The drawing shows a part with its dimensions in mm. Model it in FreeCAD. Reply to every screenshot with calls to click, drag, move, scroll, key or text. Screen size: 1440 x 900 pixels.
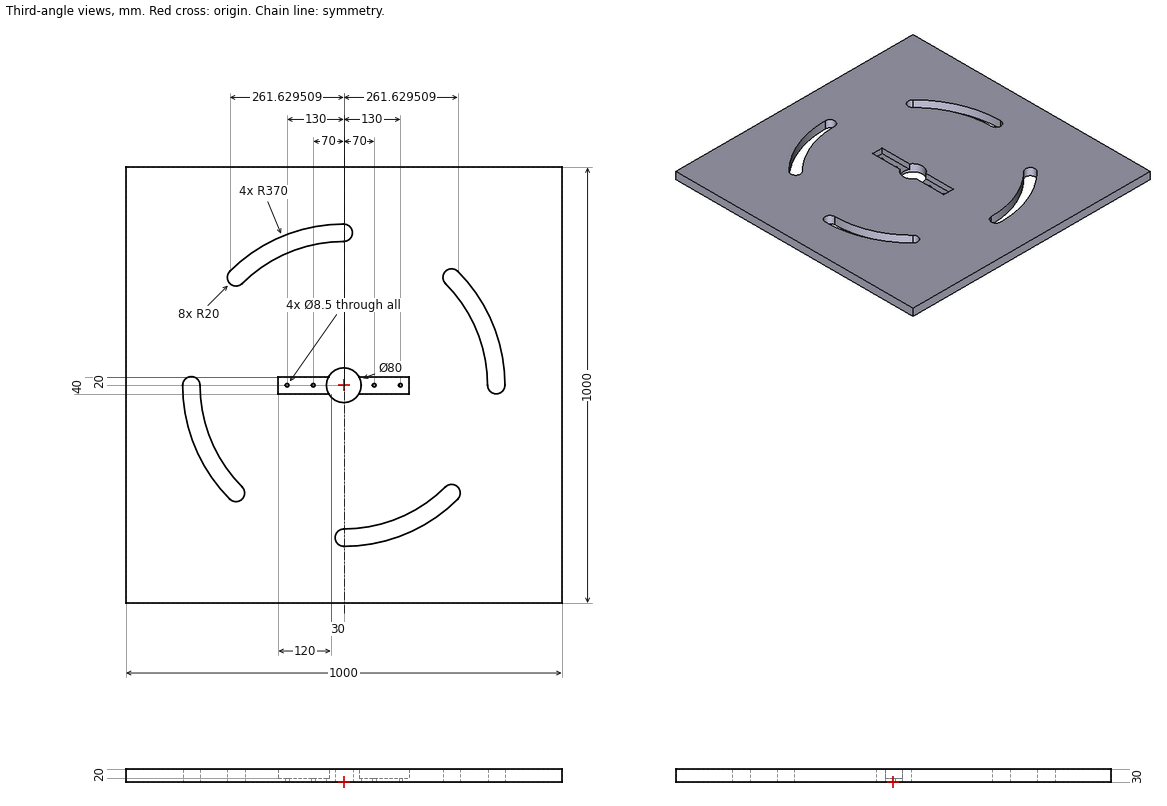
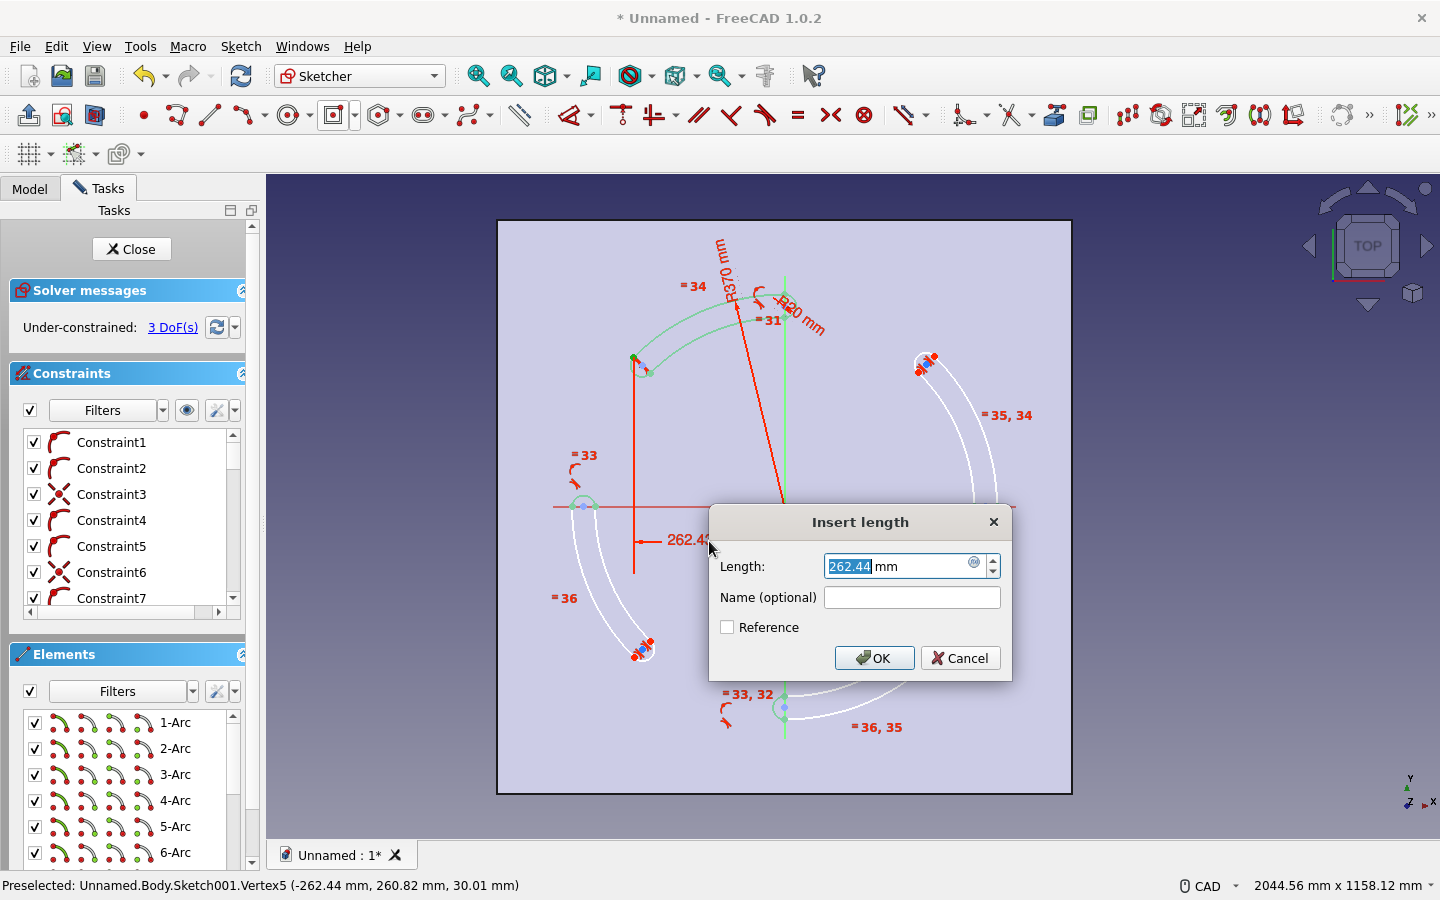
text(261.629509)
key(Return)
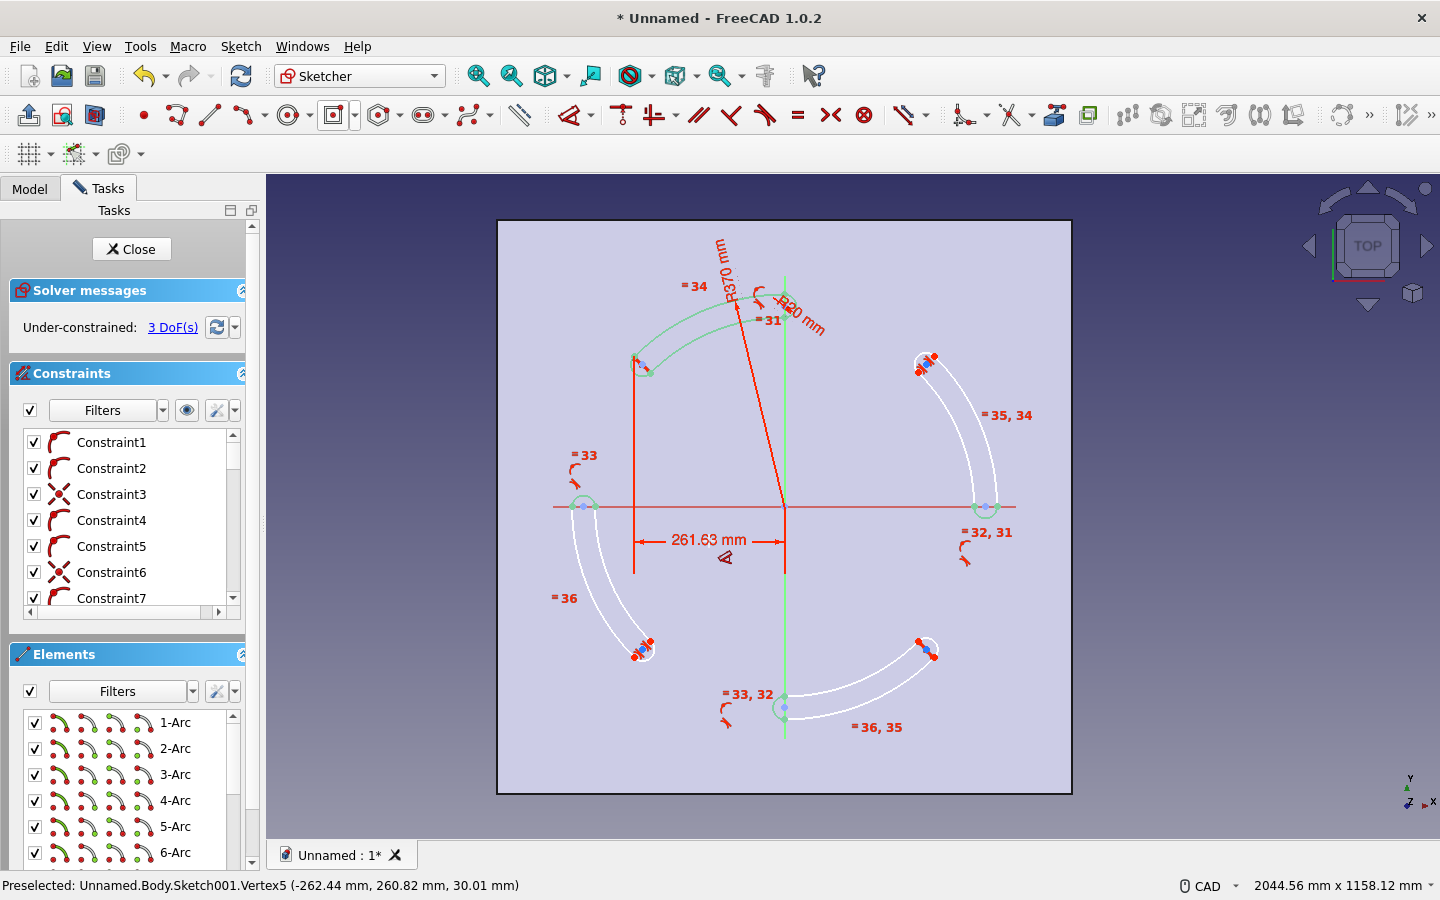
click(934, 356)
click(894, 322)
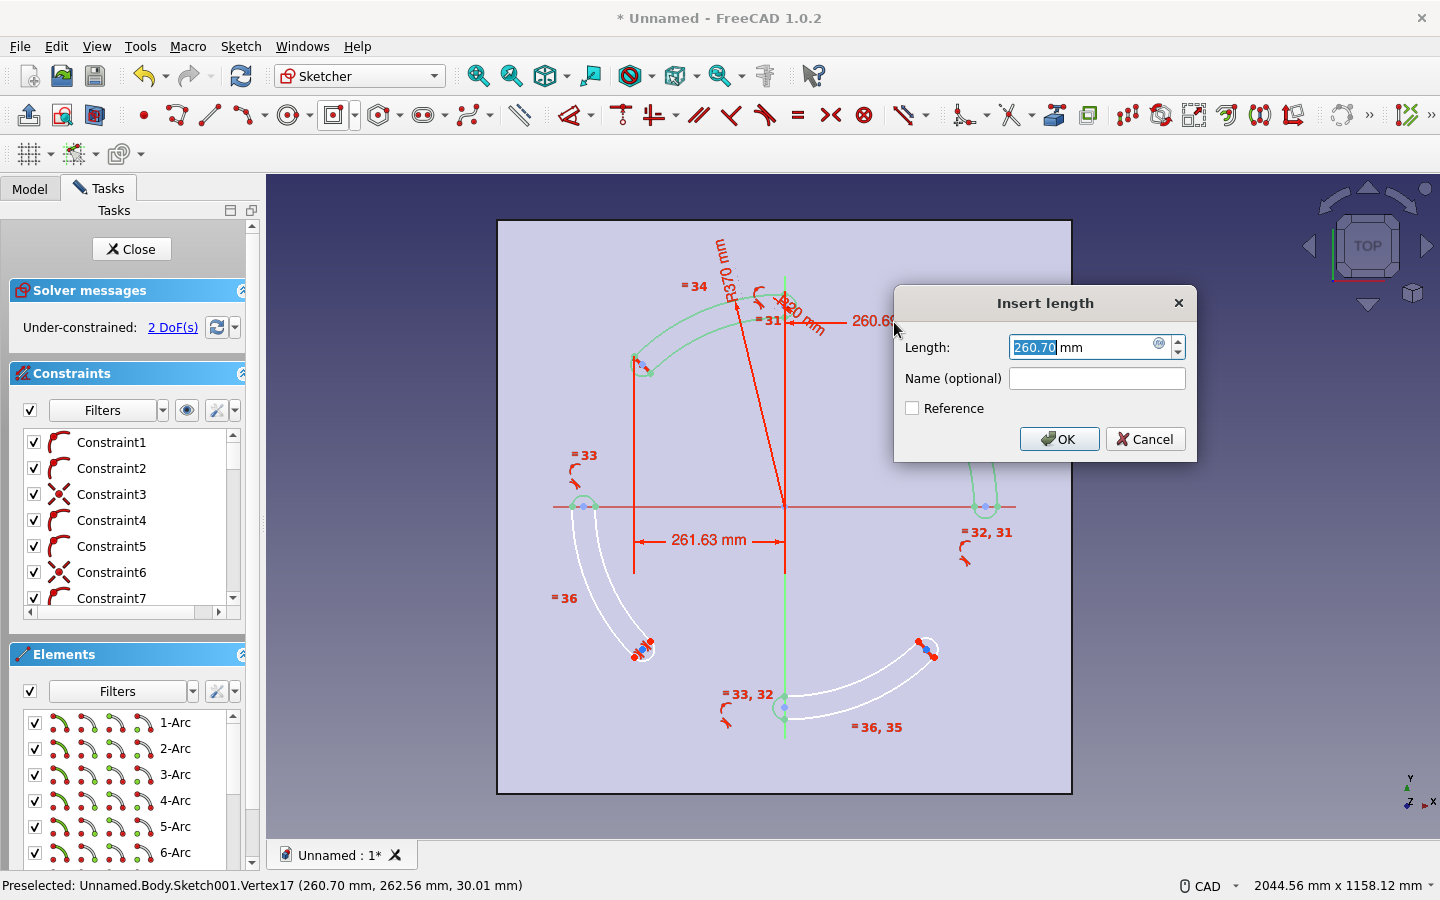
text(261.629509)
key(Return)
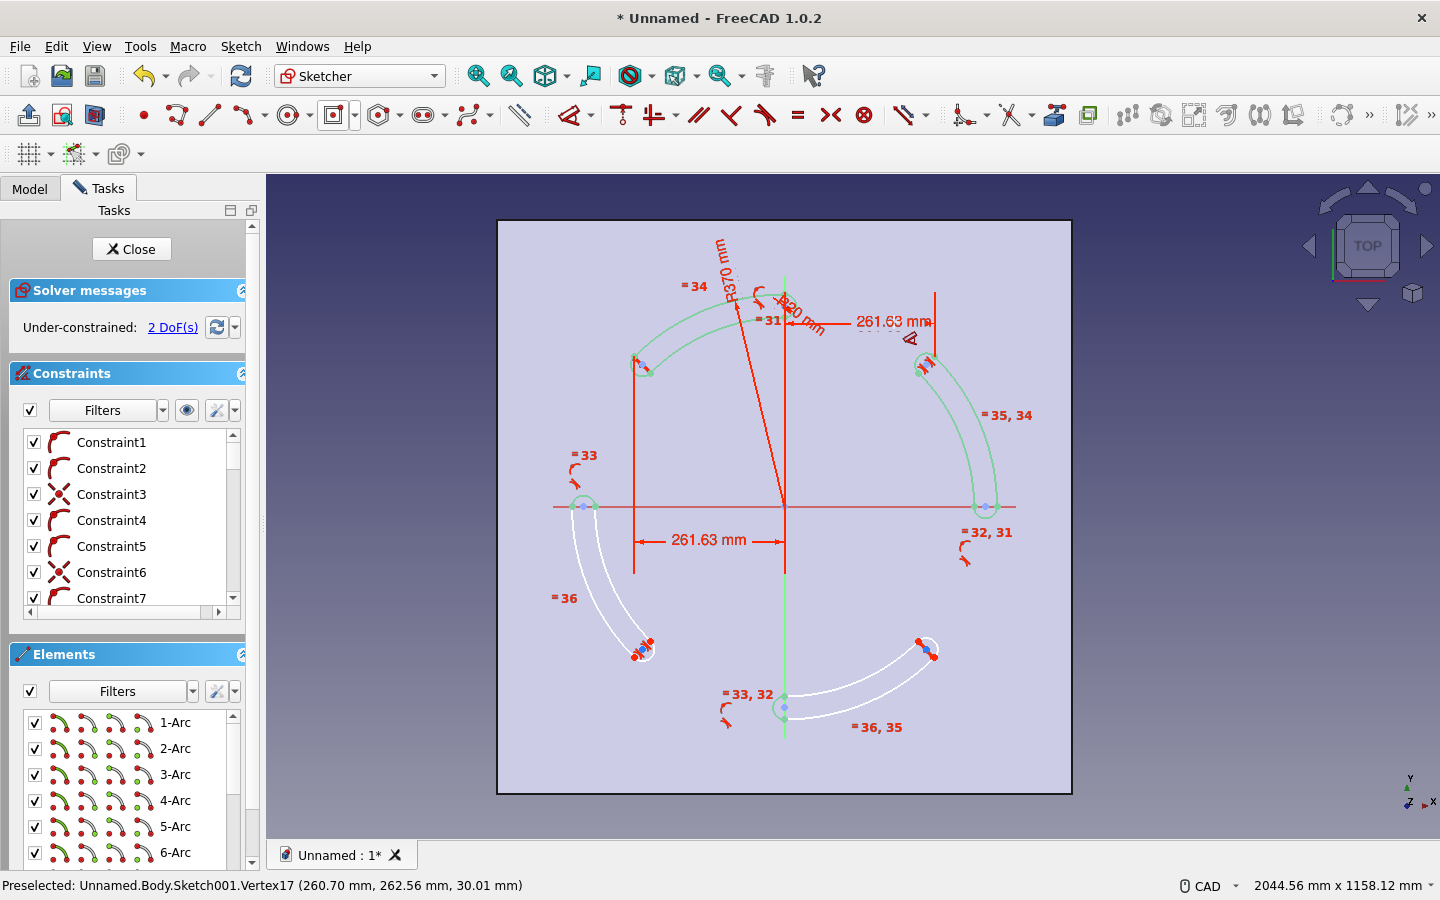
click(934, 658)
click(859, 473)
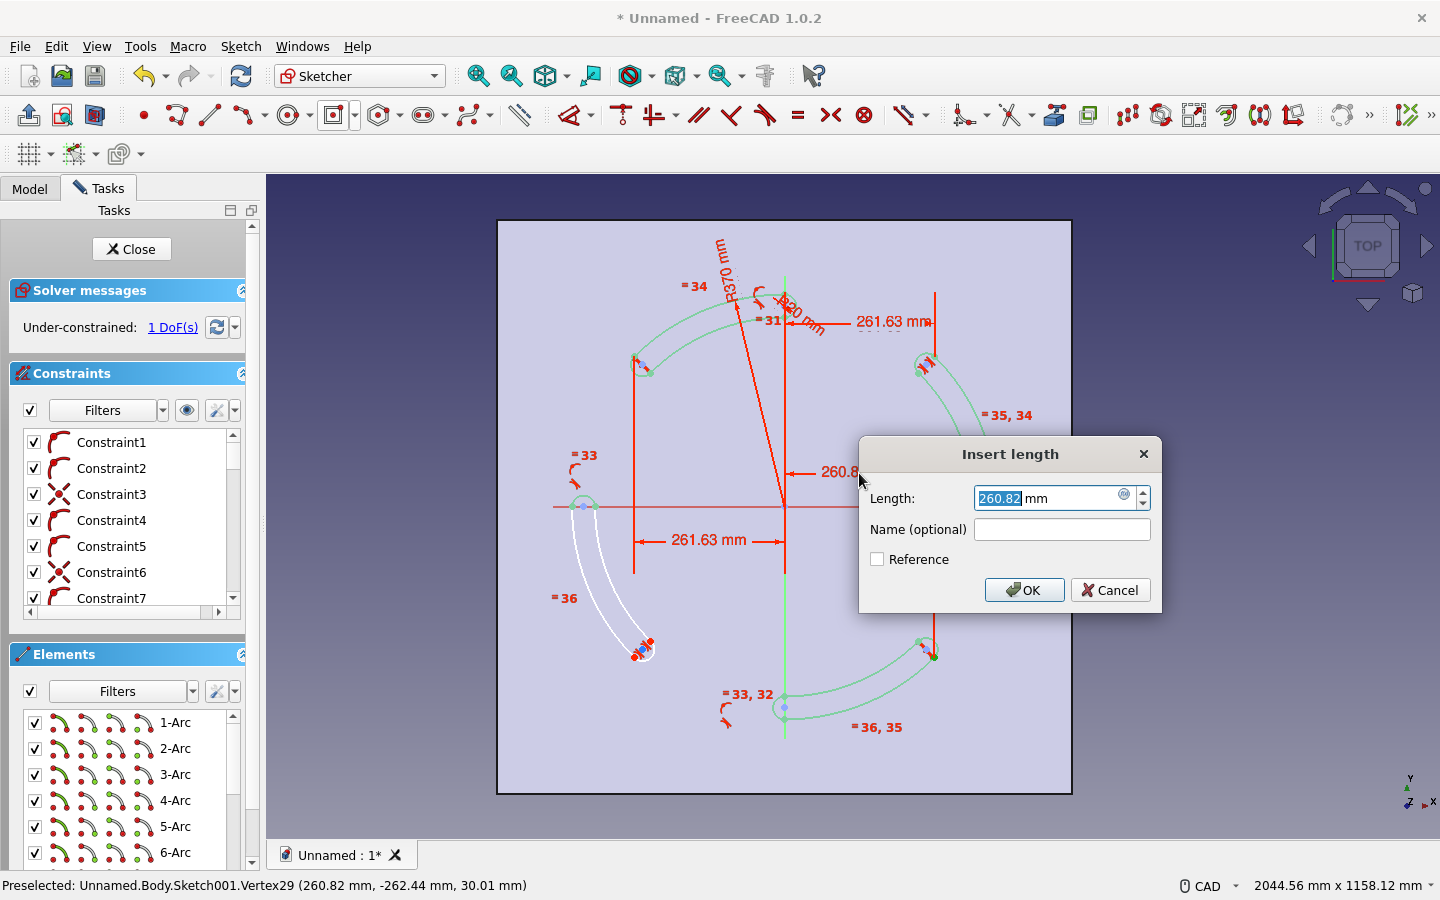
text(261.629509)
key(Return)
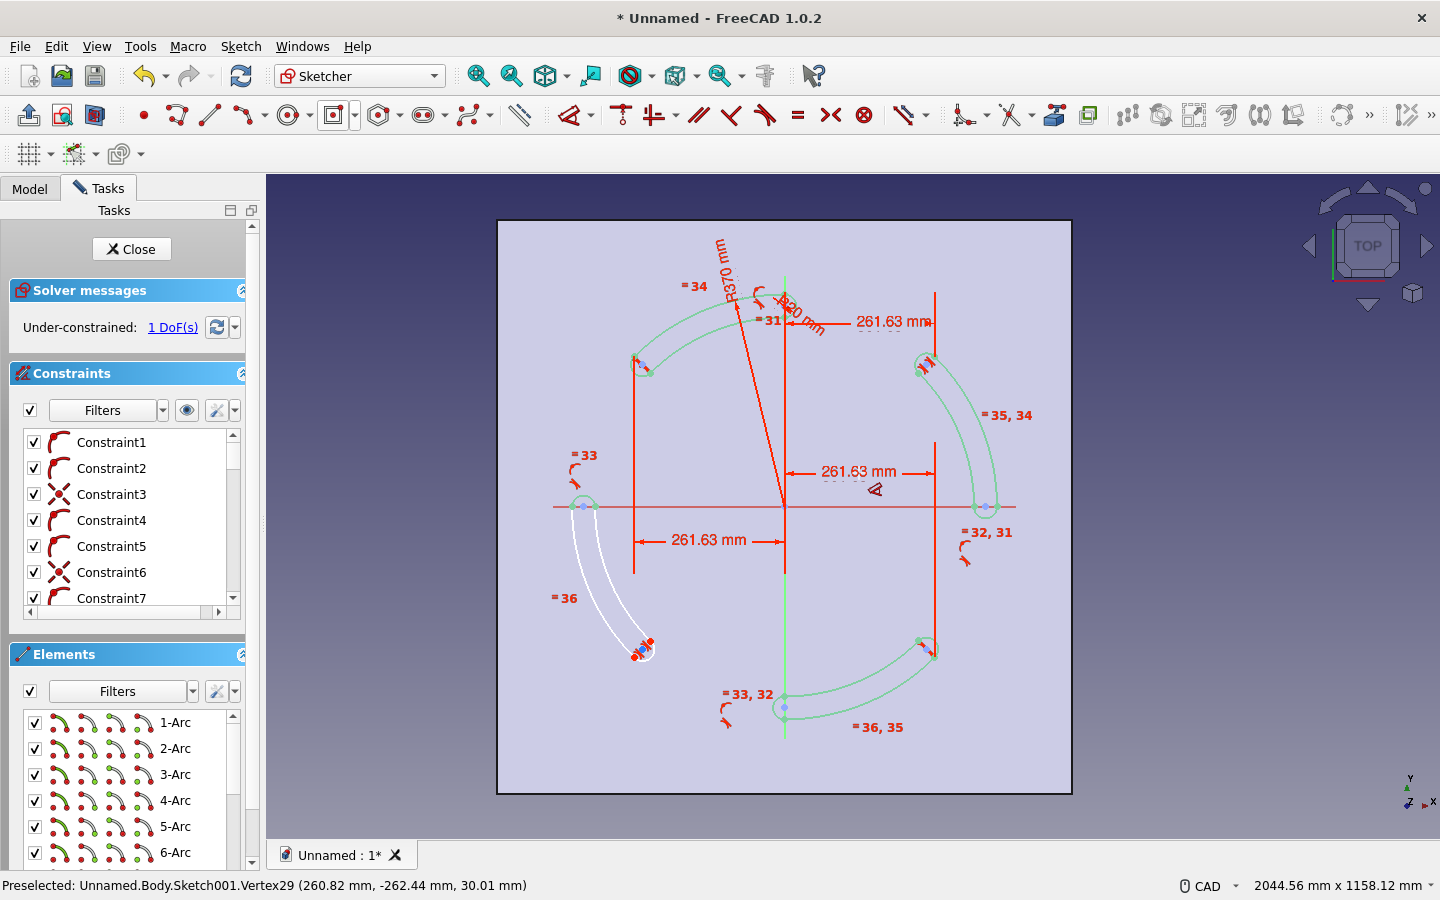
click(635, 658)
click(710, 692)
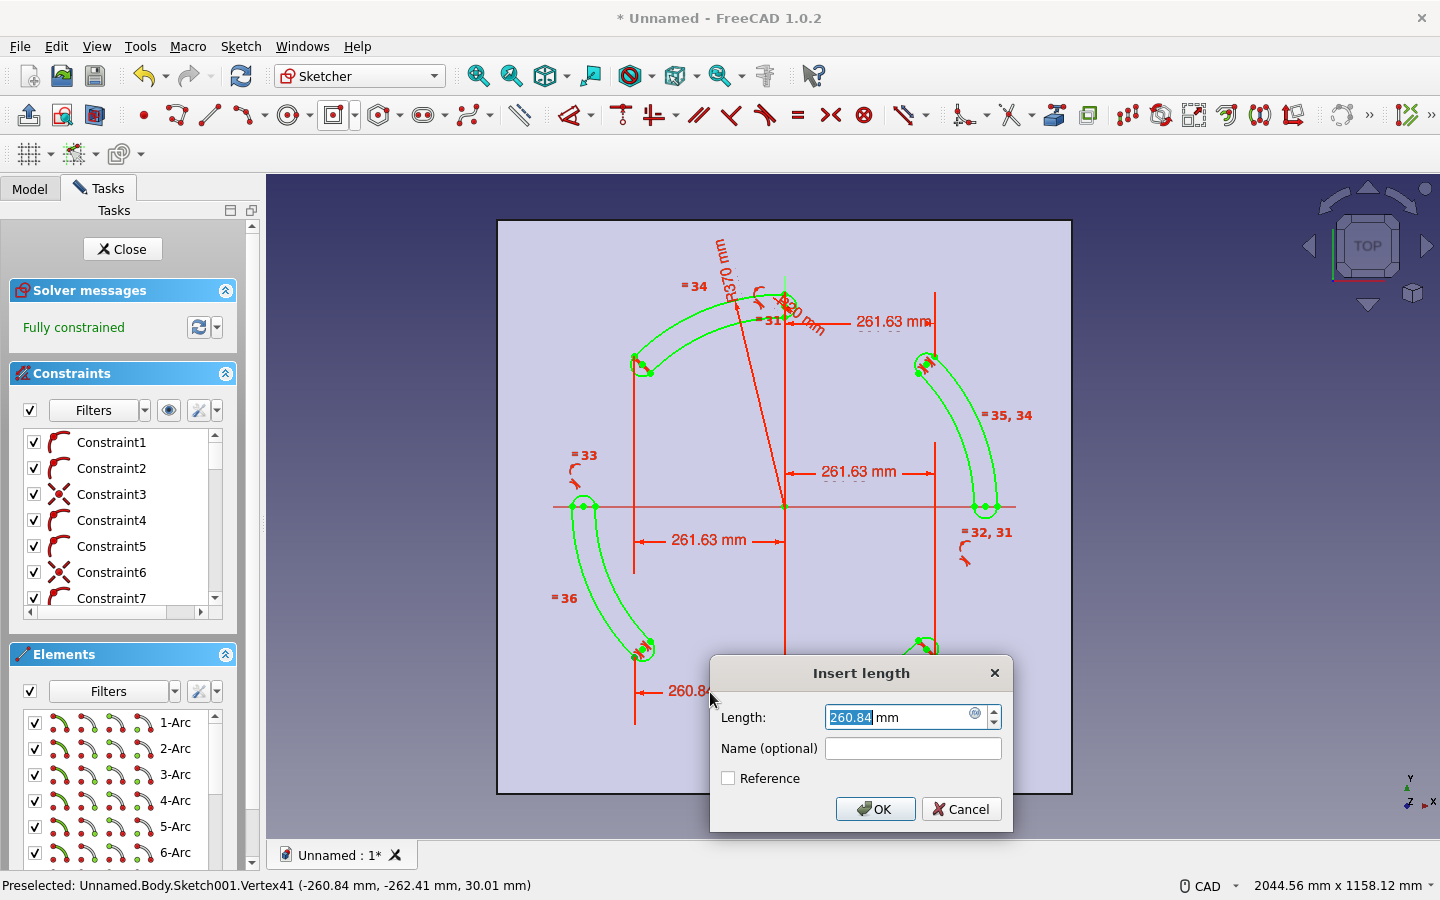
text(261.629509)
key(Return)
key(Escape)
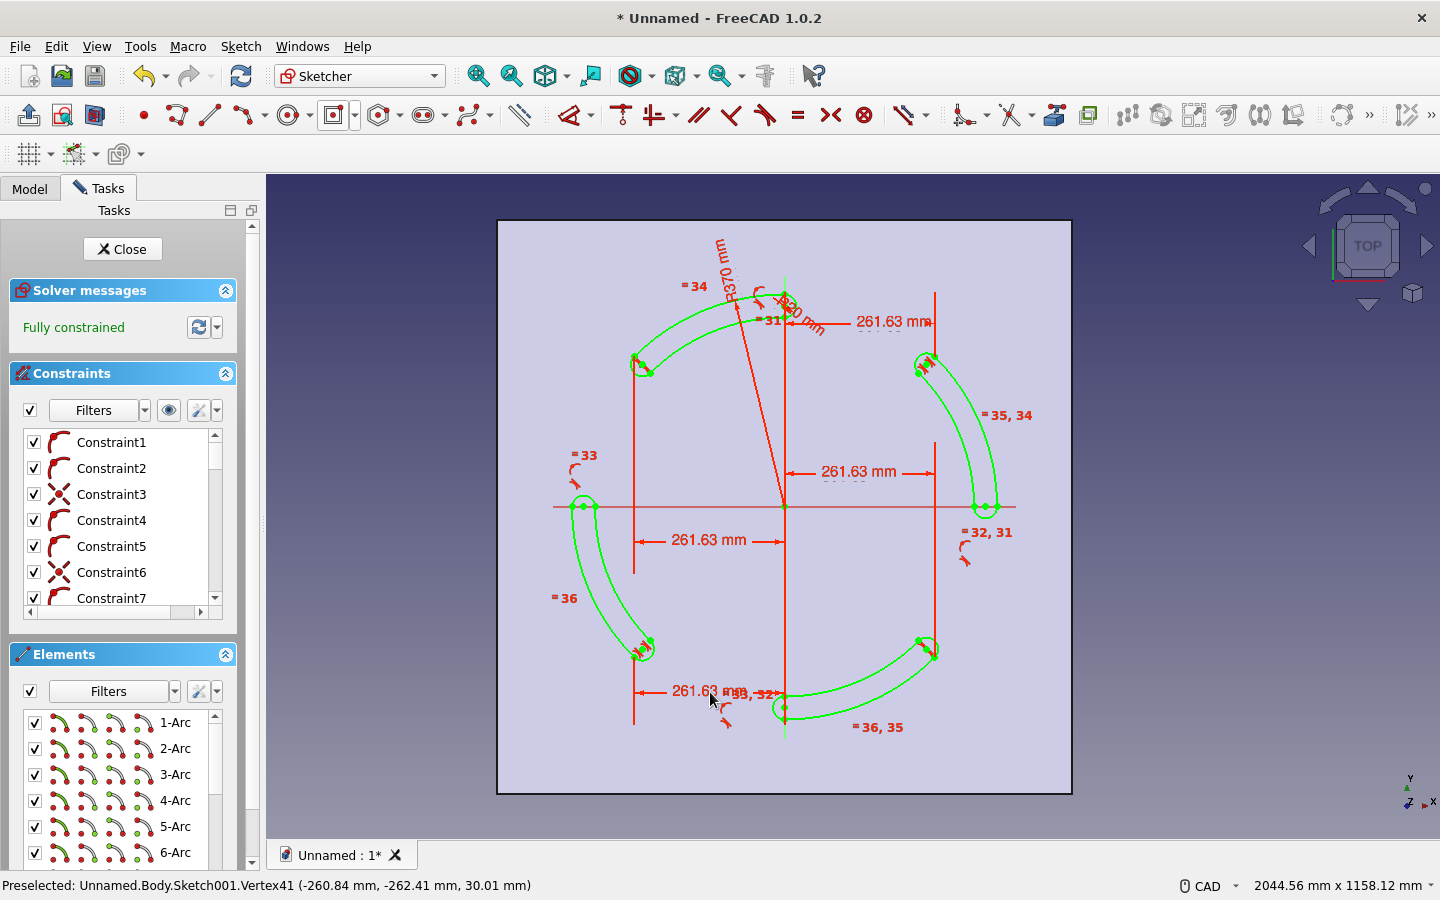
click(123, 249)